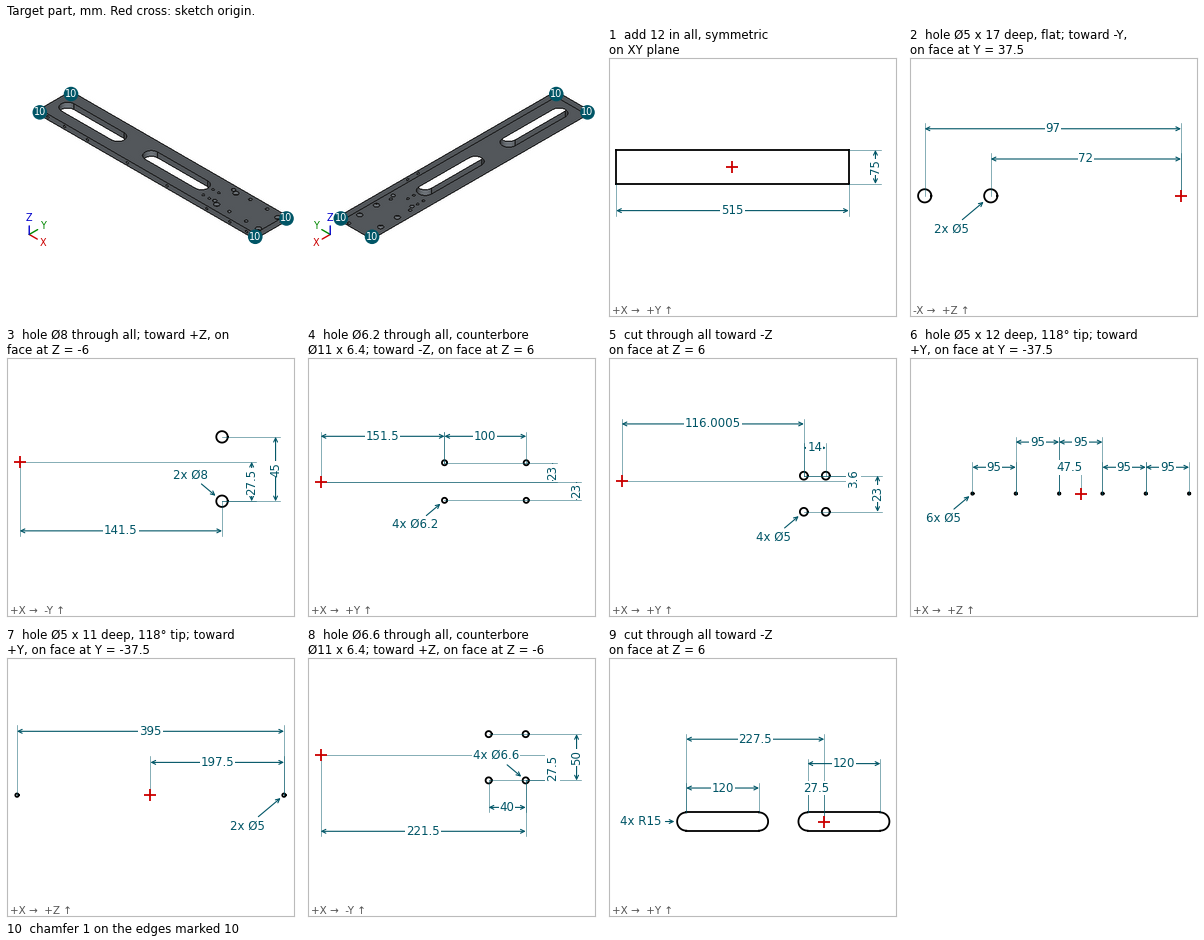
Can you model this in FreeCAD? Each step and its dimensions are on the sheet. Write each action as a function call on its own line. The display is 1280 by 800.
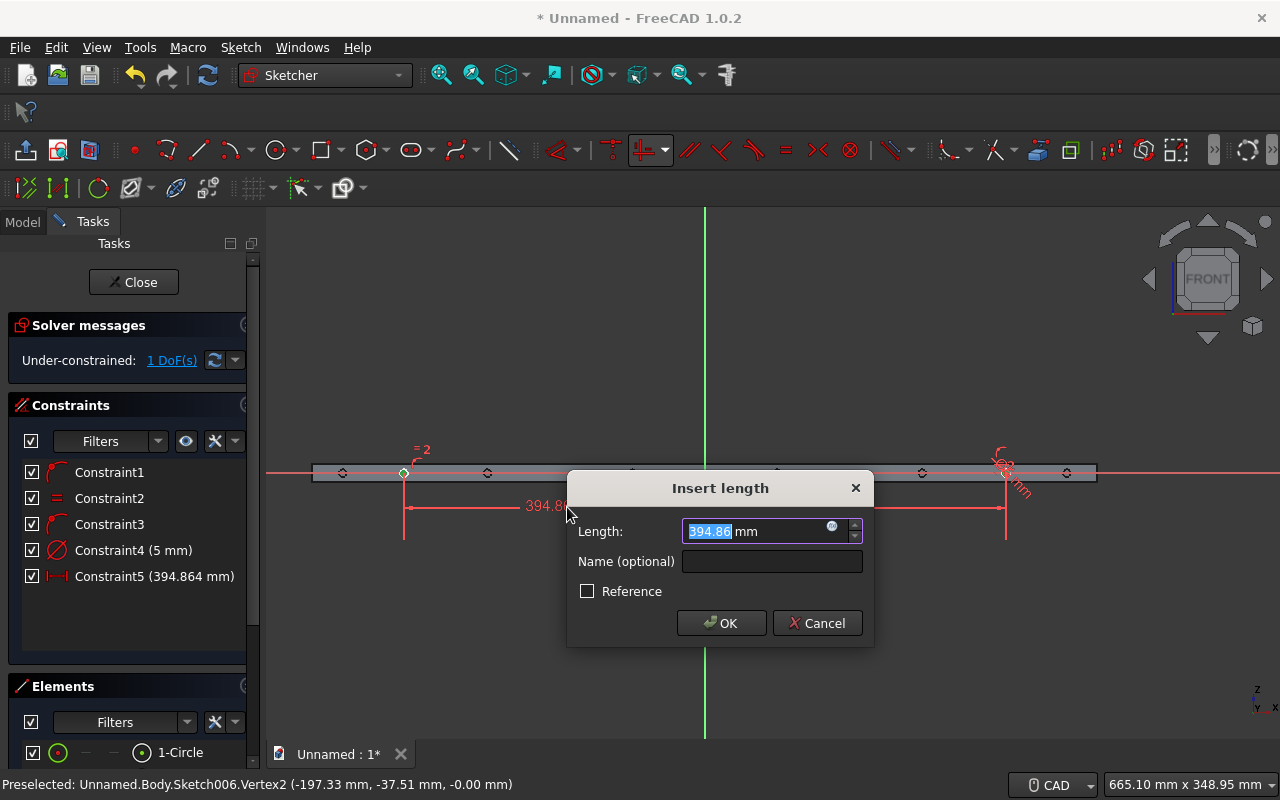
text(395)
key(Return)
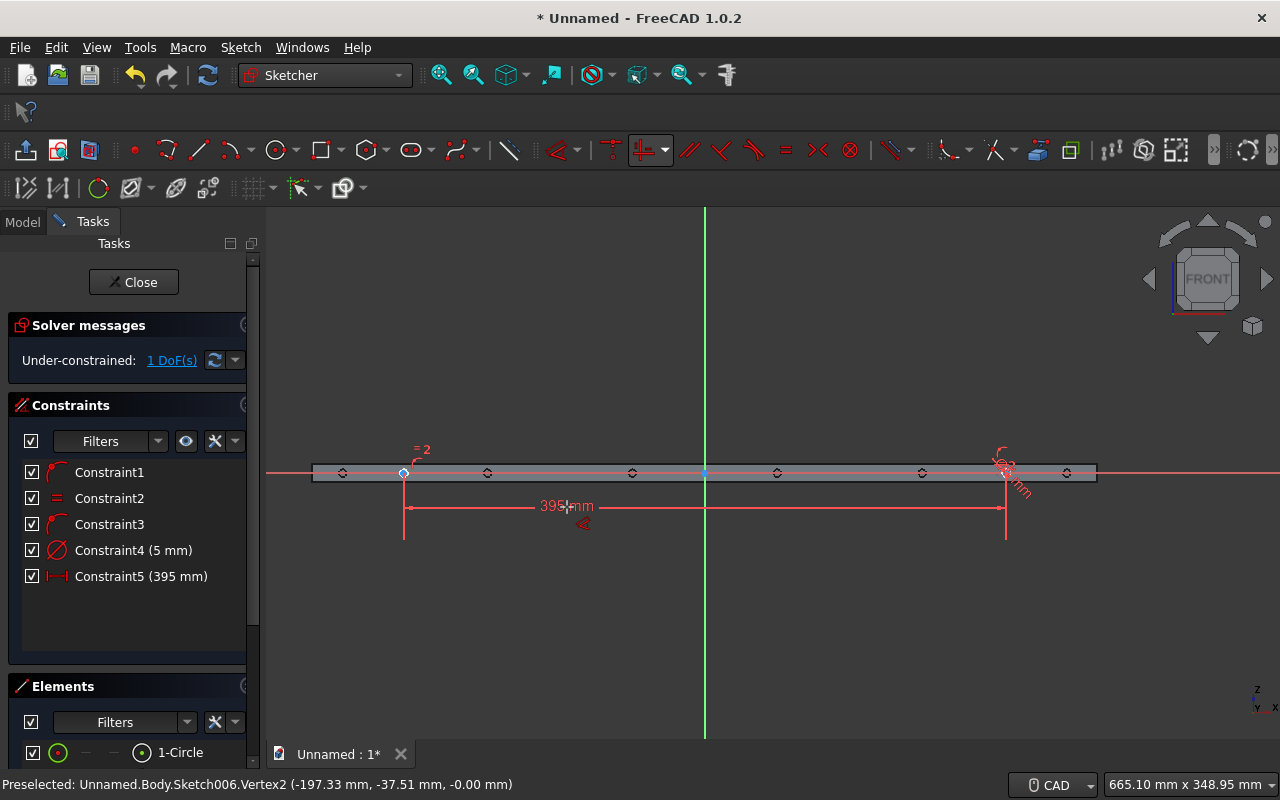
click(1006, 473)
click(855, 507)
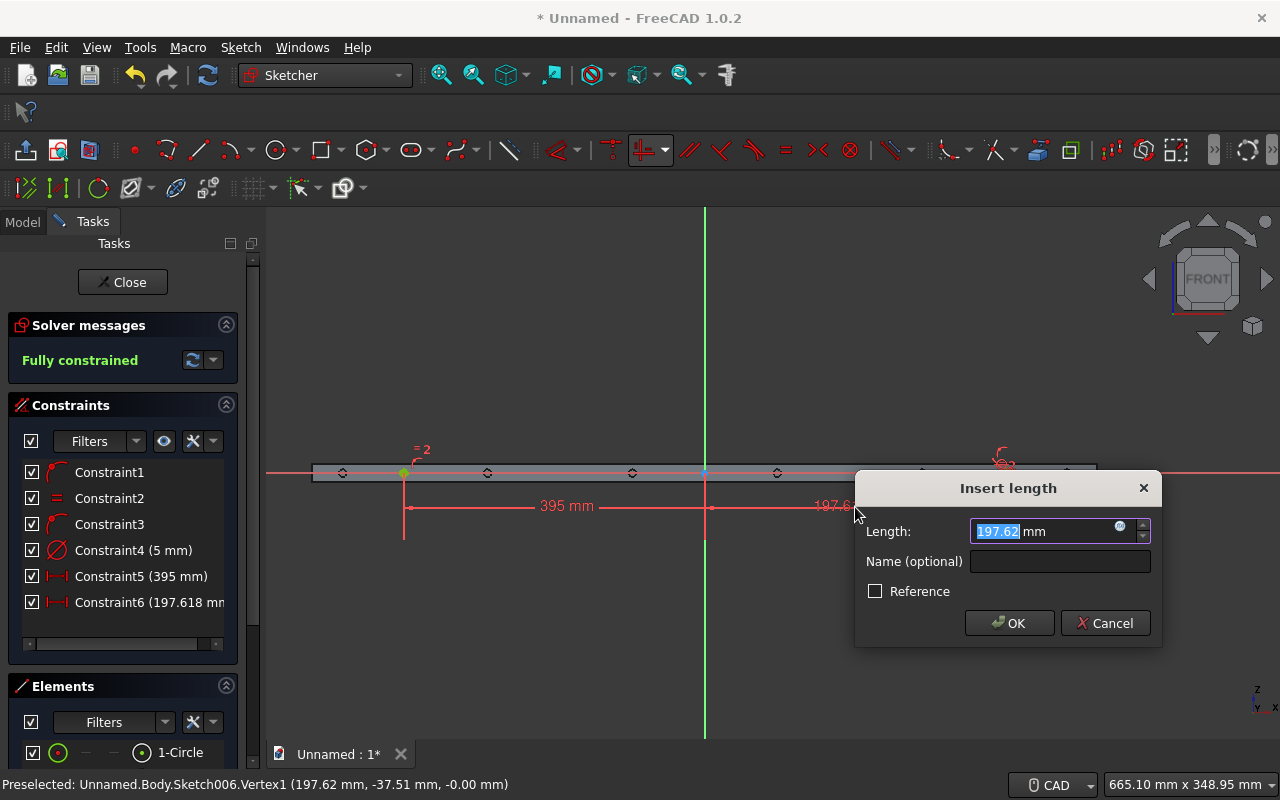
text(197.5)
key(Return)
key(Escape)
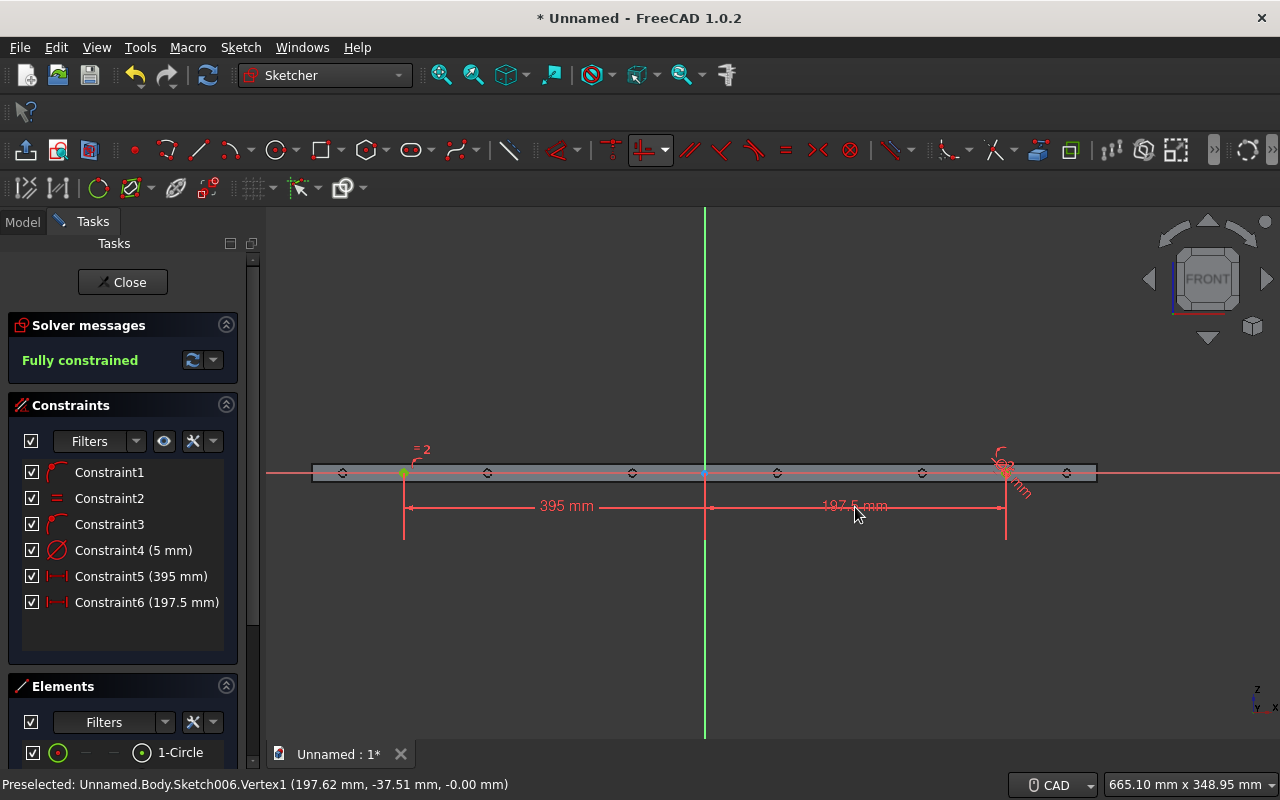
click(123, 282)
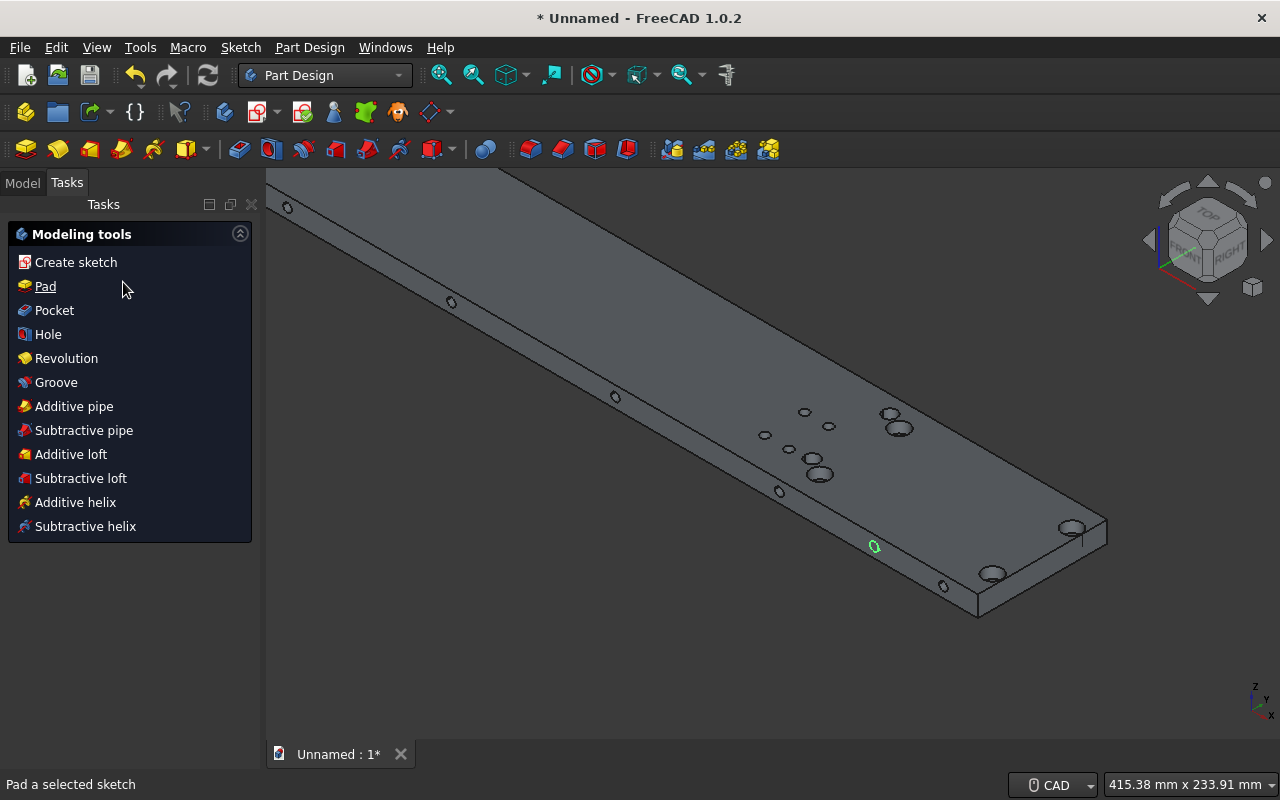
click(272, 150)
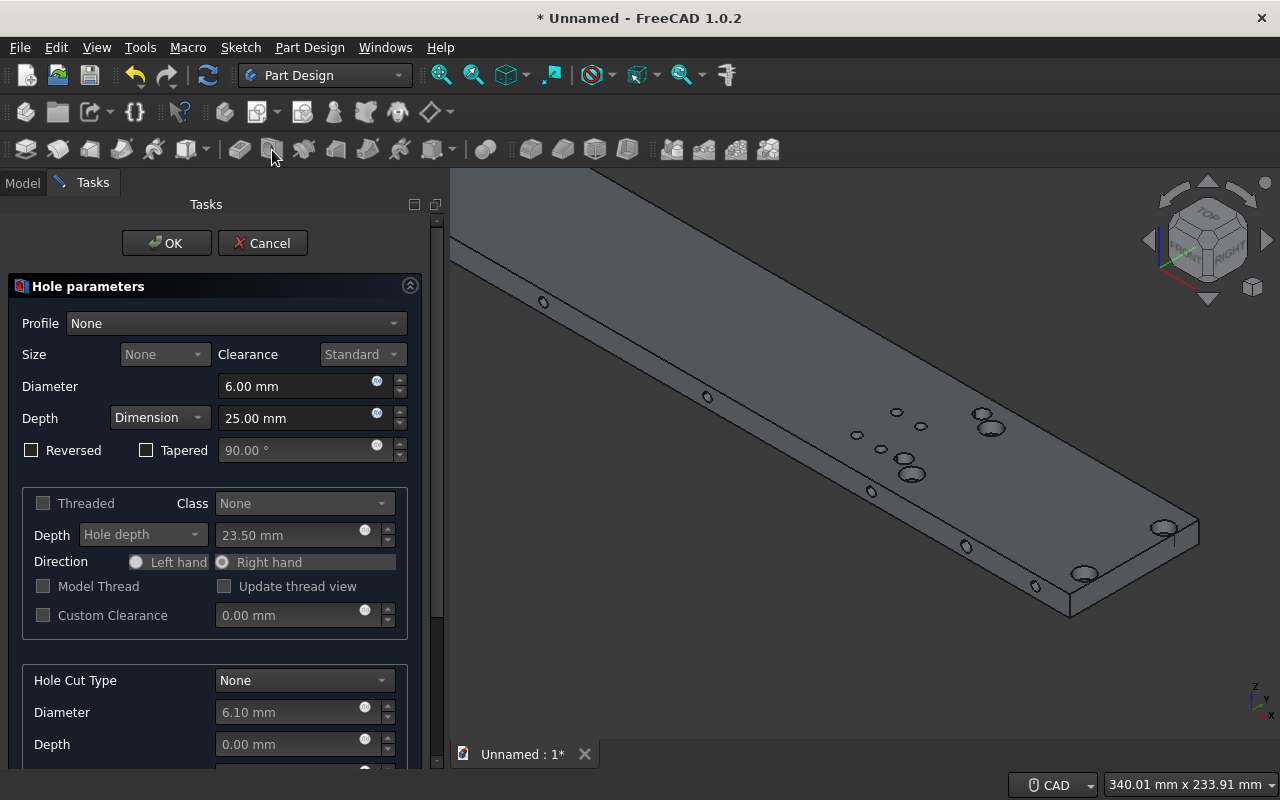
triple_click(305, 386)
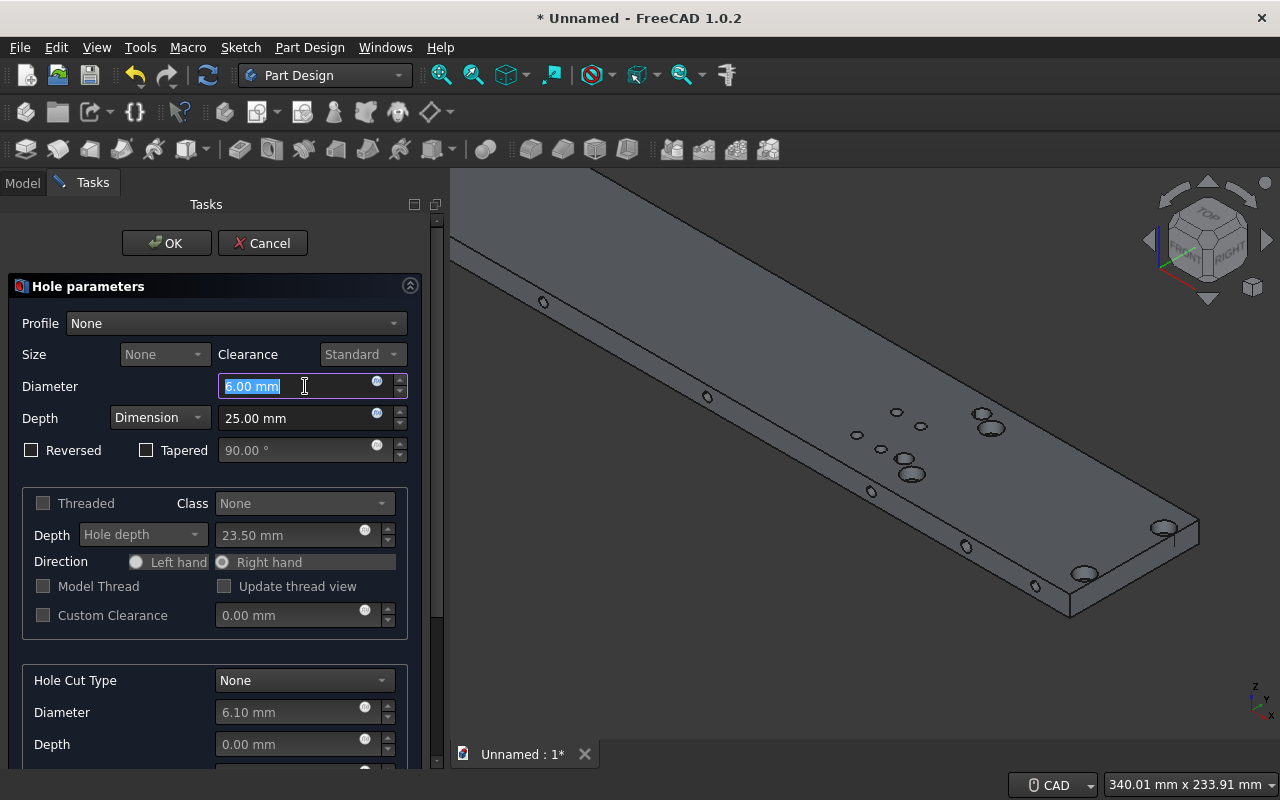
text(5)
key(Tab)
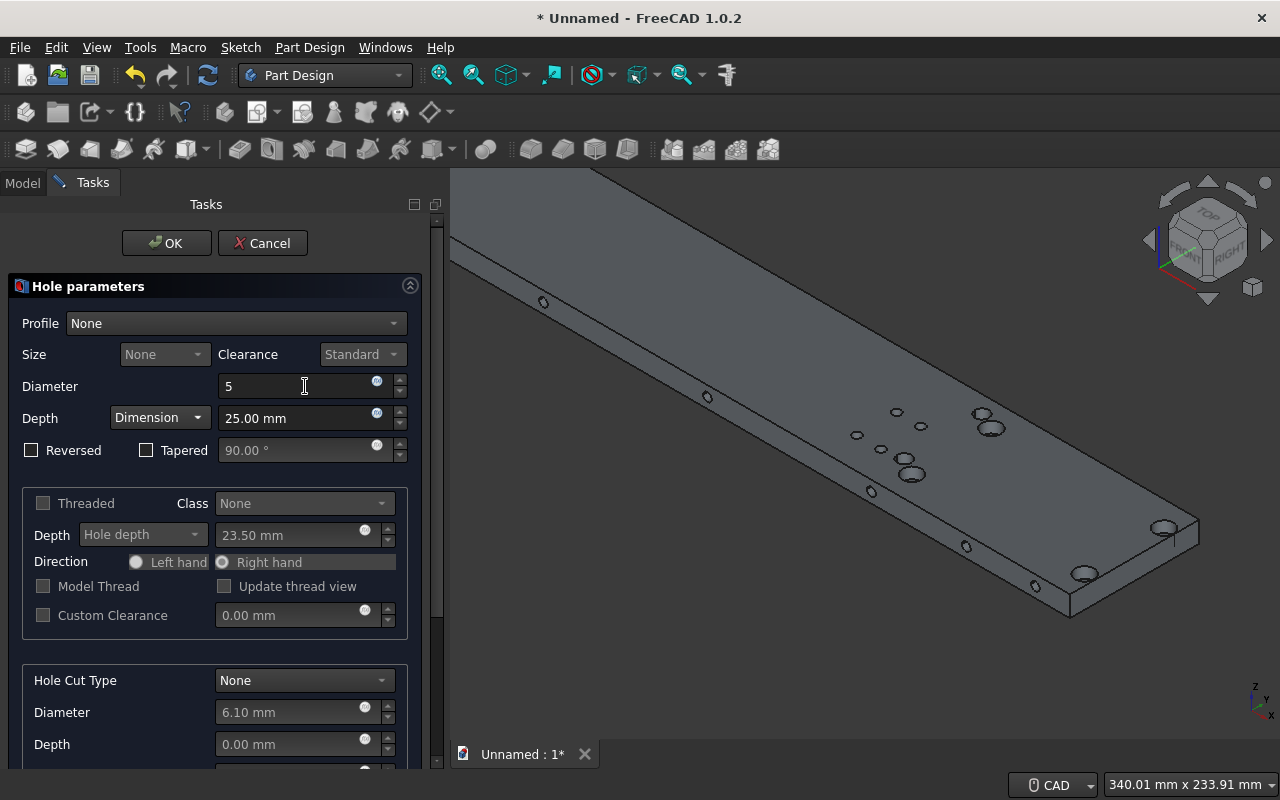
triple_click(305, 418)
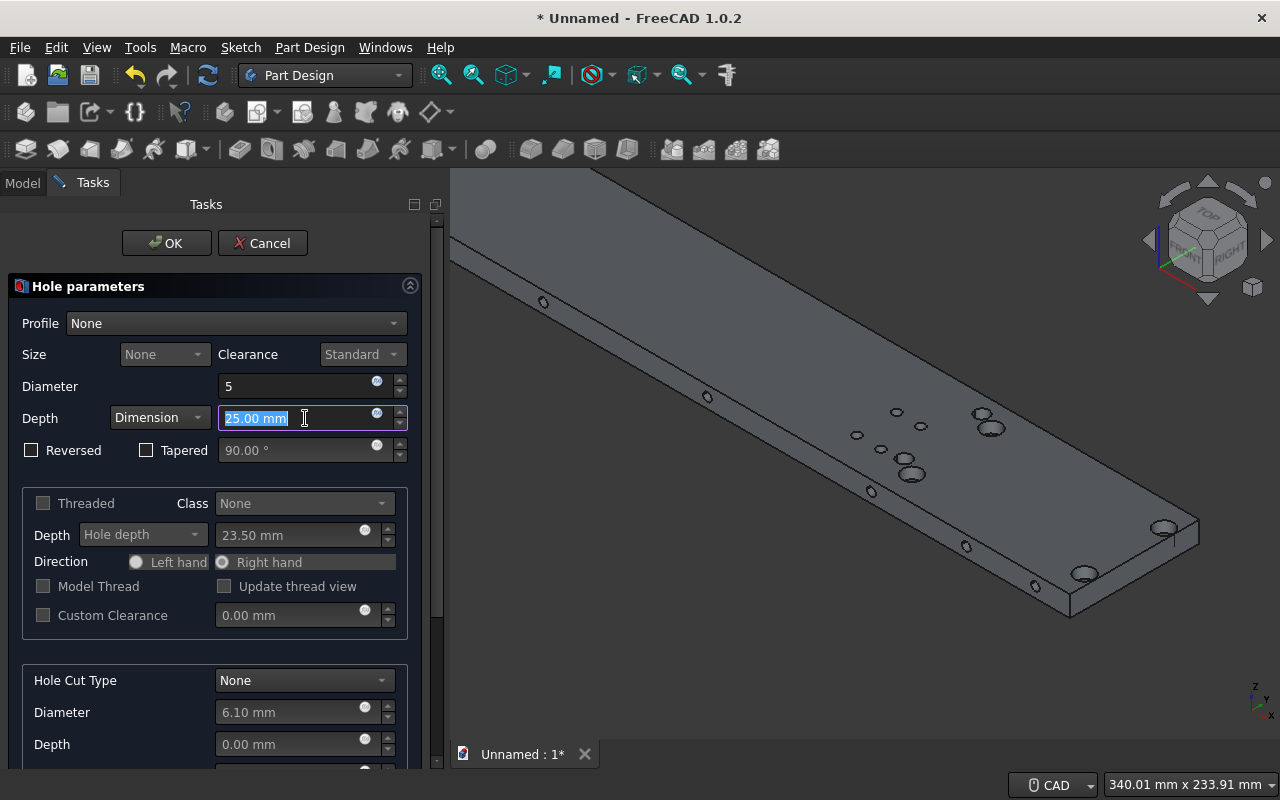
text(11)
key(Tab)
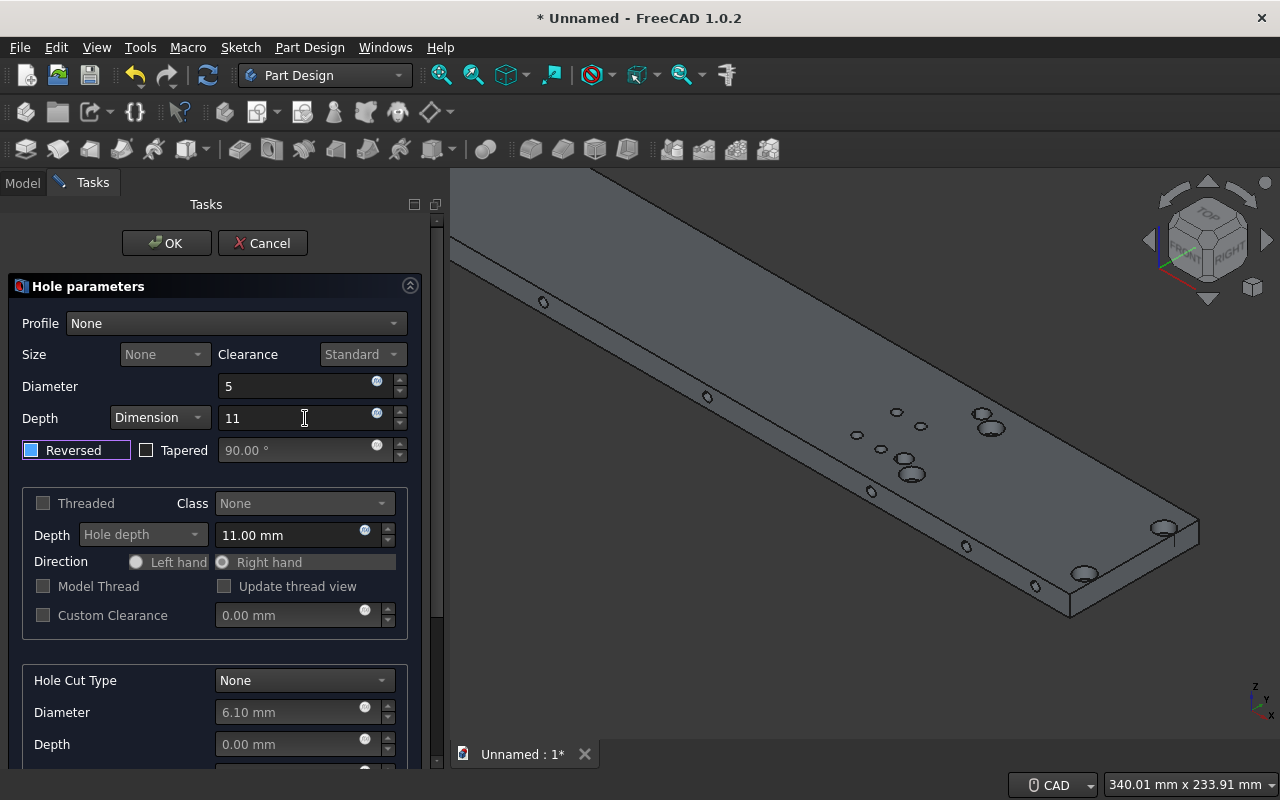
click(167, 243)